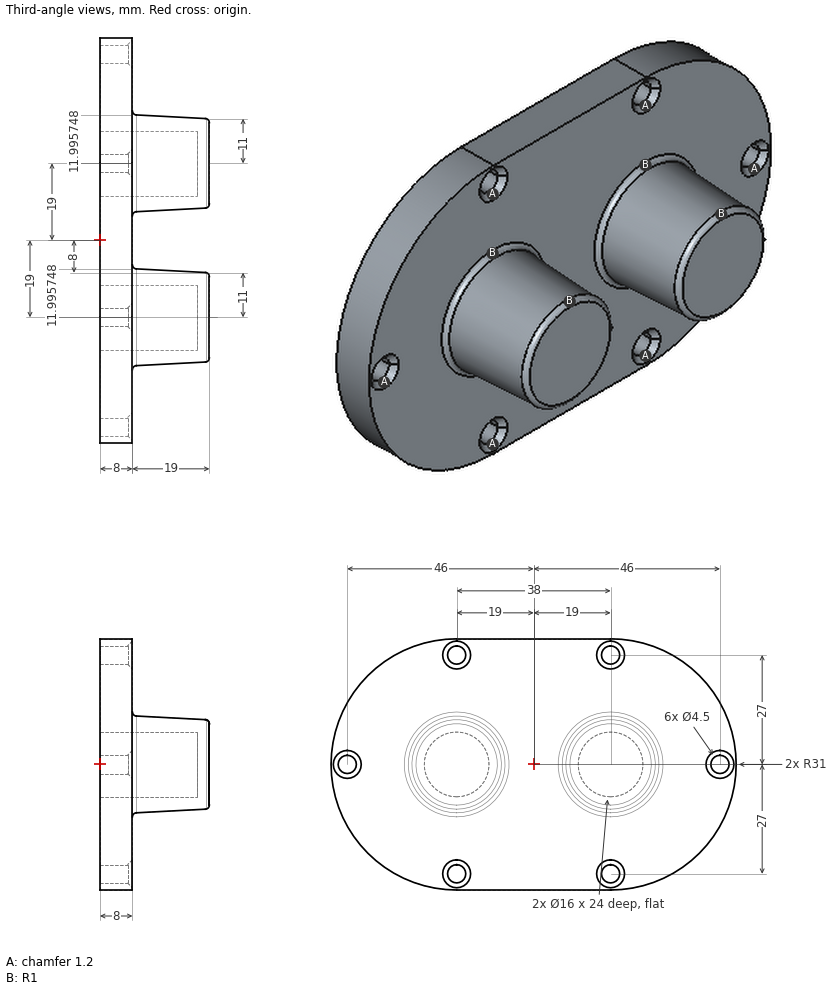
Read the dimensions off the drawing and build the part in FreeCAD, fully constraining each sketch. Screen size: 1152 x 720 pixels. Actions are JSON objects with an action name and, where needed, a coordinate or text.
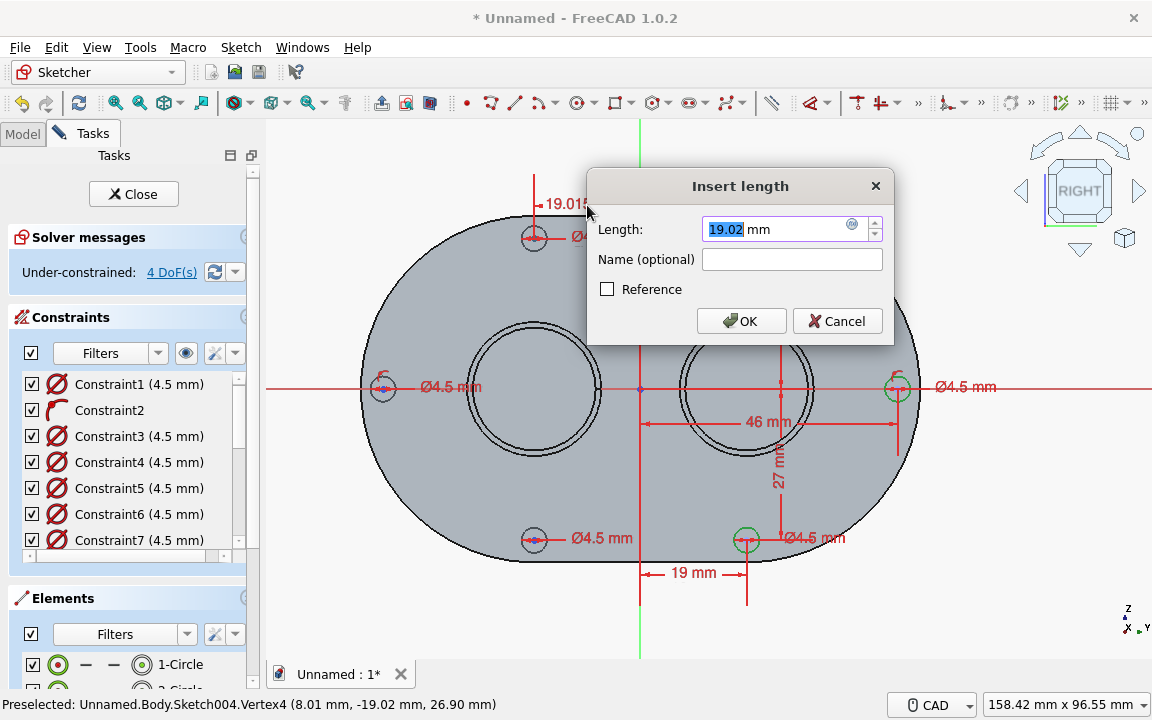
{"action": "type", "text": "19"}
{"action": "key", "text": "Return"}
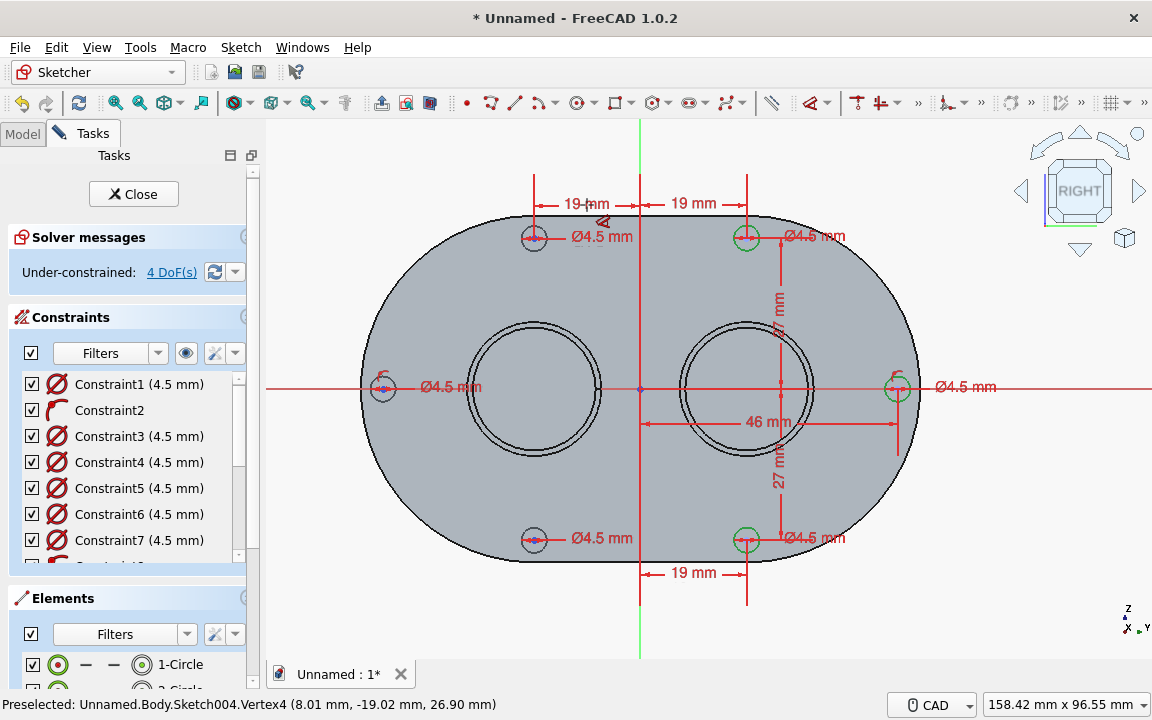
{"action": "left_click", "coordinate": [534, 239]}
{"action": "left_click", "coordinate": [500, 314]}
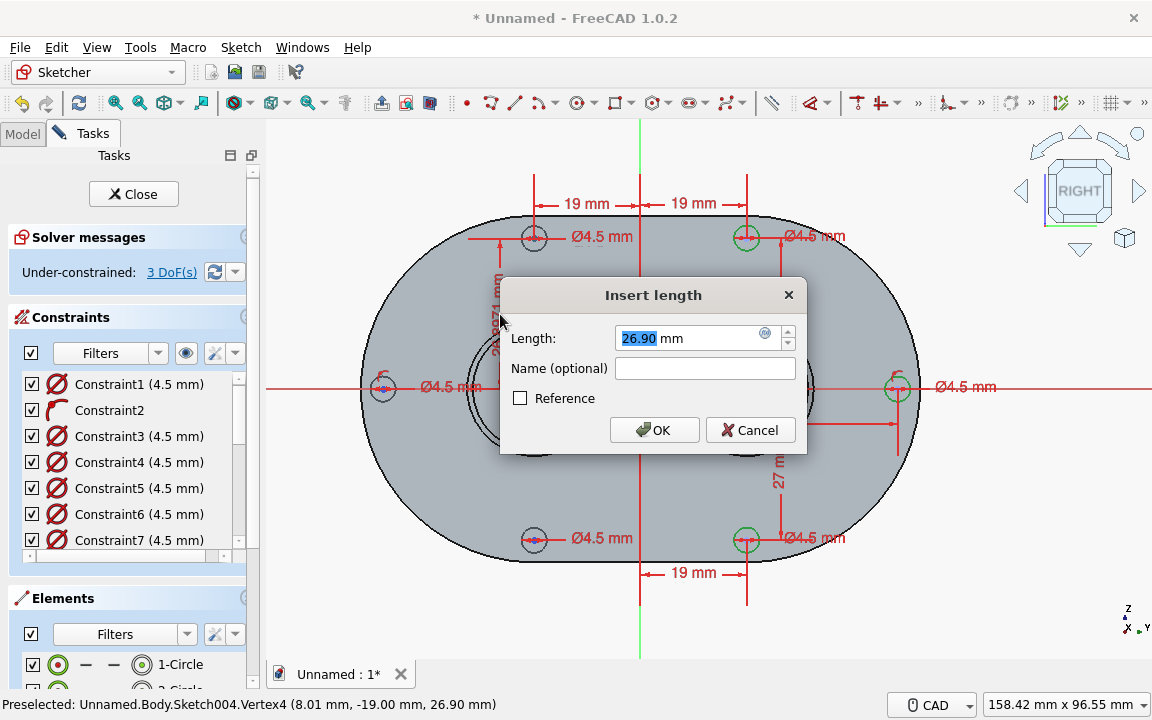
{"action": "type", "text": "27"}
{"action": "key", "text": "Return"}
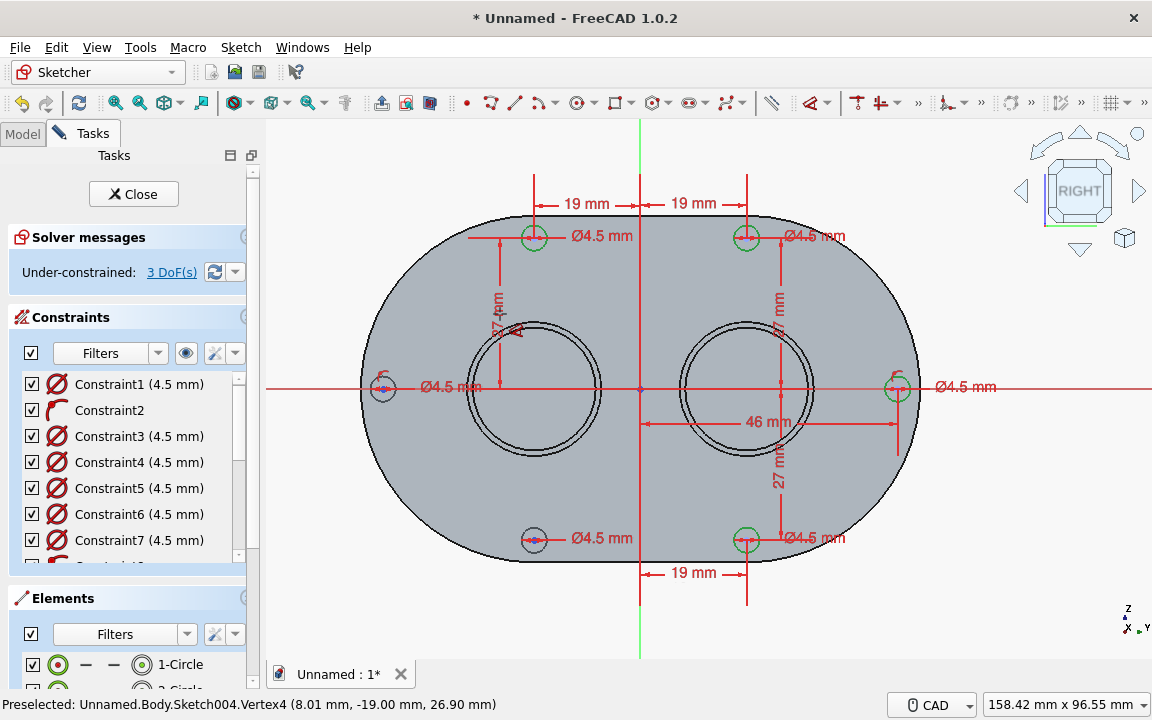
{"action": "left_click", "coordinate": [534, 540]}
{"action": "left_click", "coordinate": [587, 574]}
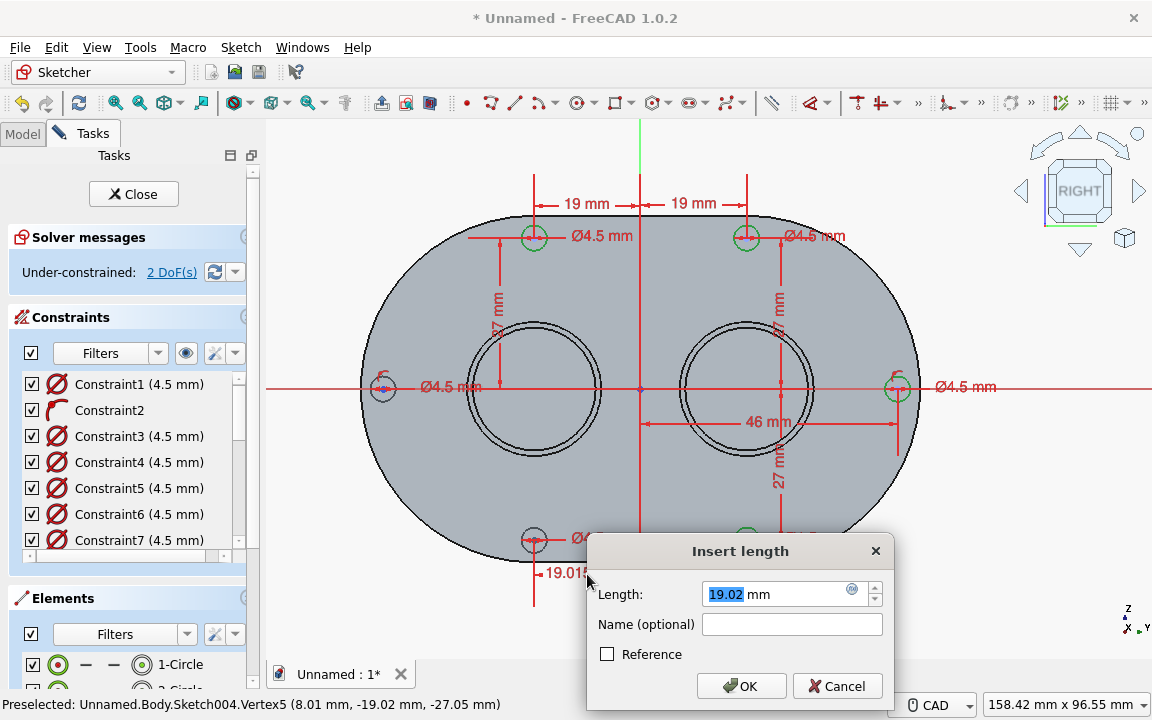
{"action": "type", "text": "19"}
{"action": "key", "text": "Return"}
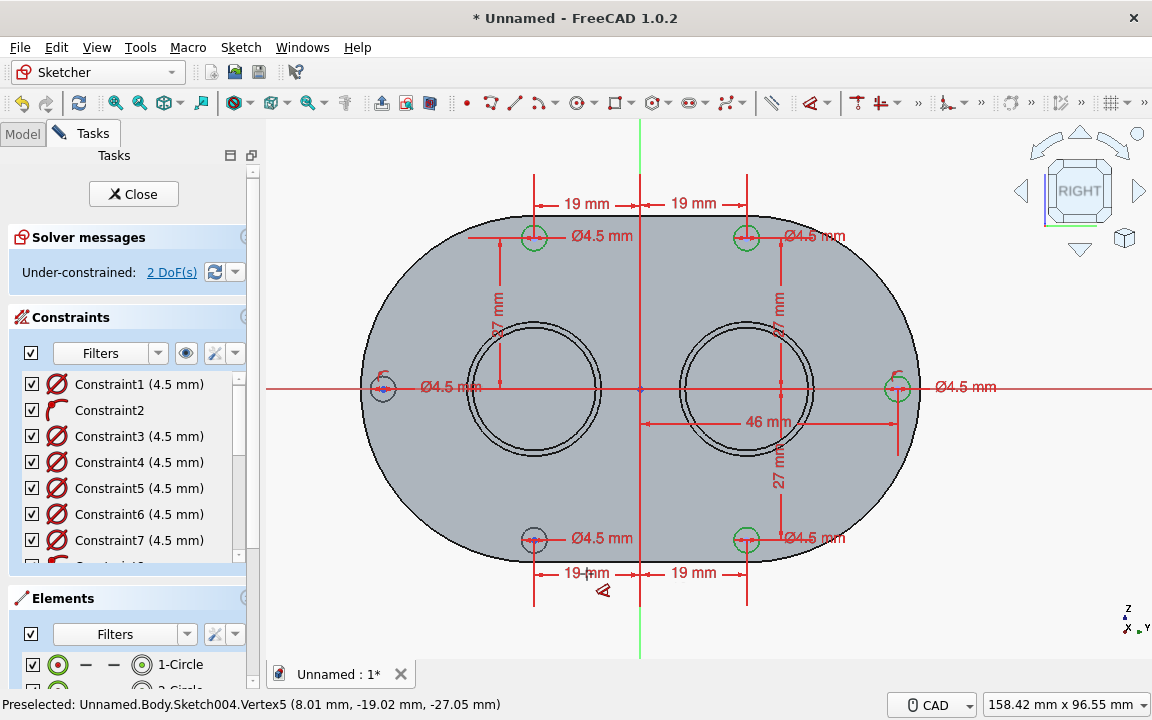
{"action": "left_click", "coordinate": [534, 540]}
{"action": "left_click", "coordinate": [500, 465]}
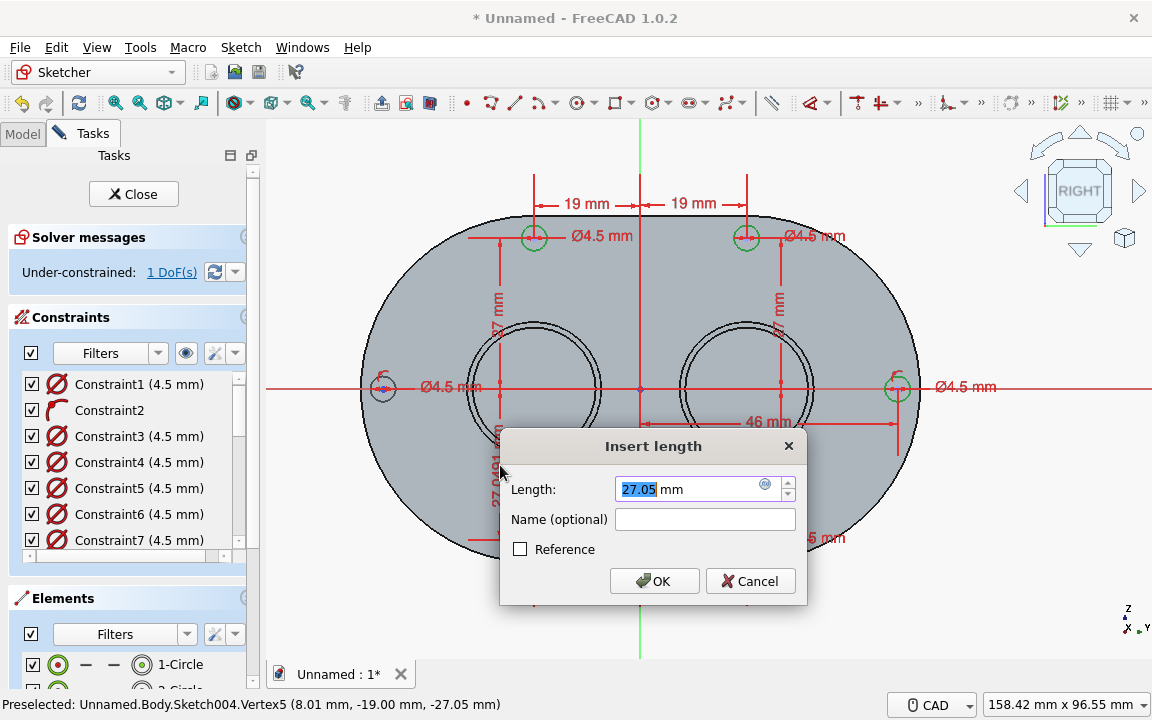
{"action": "type", "text": "27"}
{"action": "key", "text": "Return"}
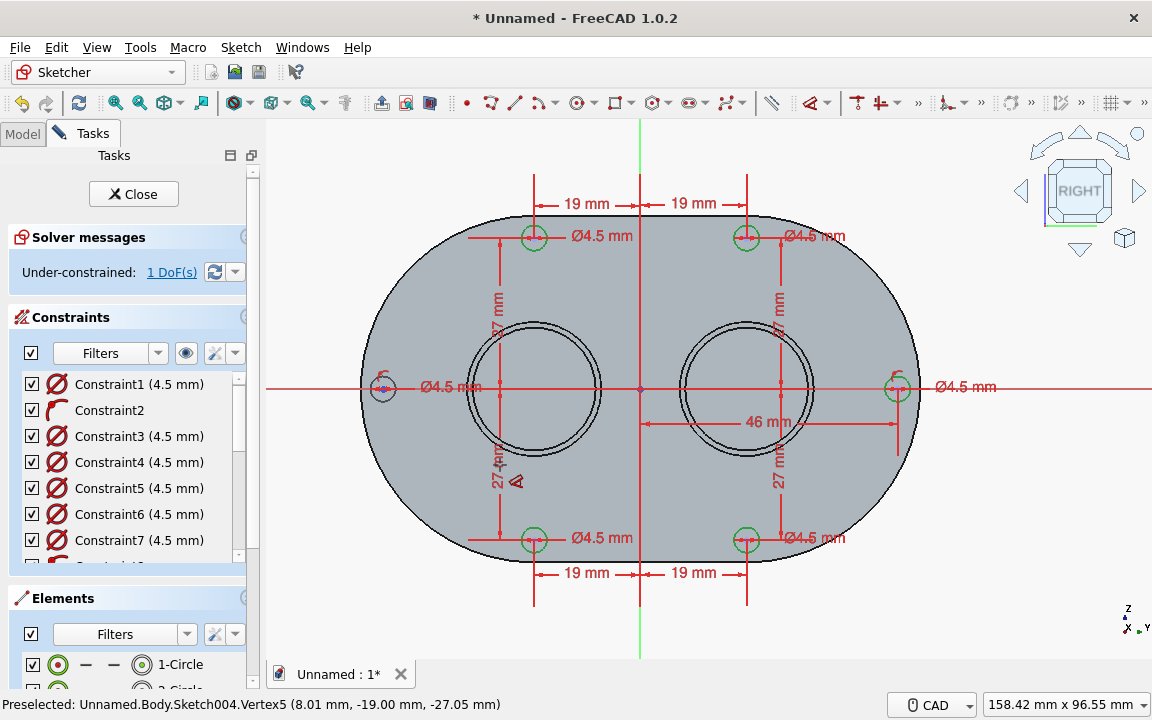
{"action": "left_click", "coordinate": [383, 389]}
{"action": "left_click", "coordinate": [512, 423]}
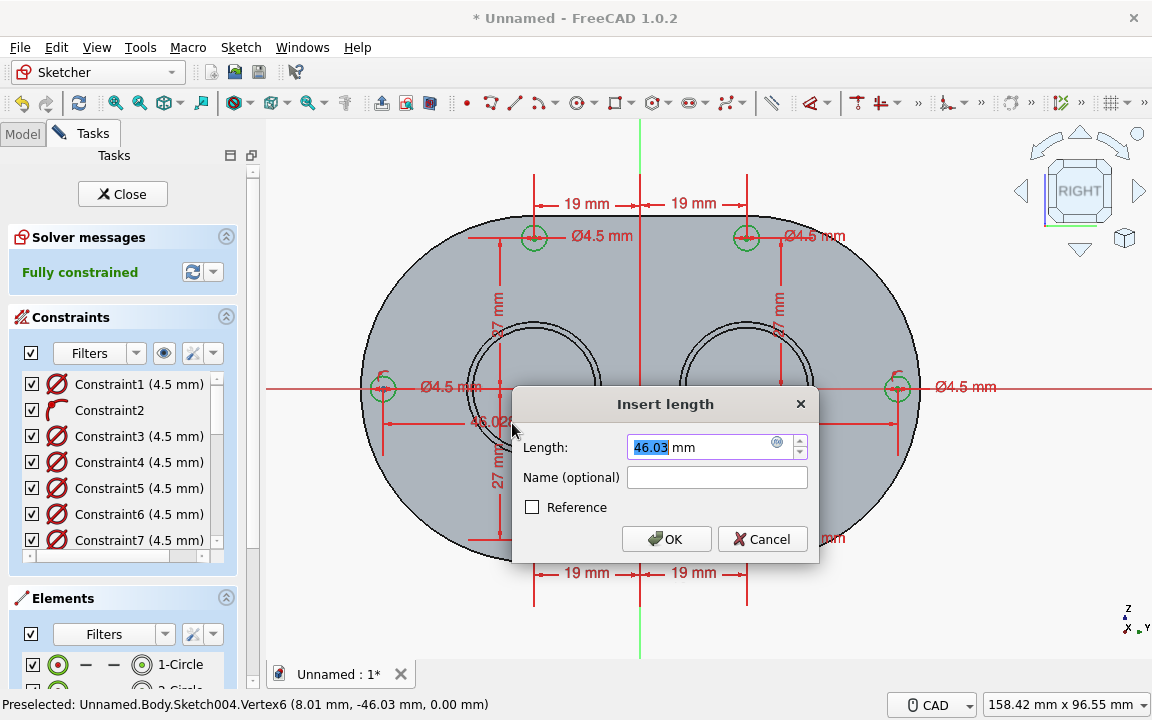
{"action": "type", "text": "46"}
{"action": "key", "text": "Return"}
{"action": "key", "text": "Escape"}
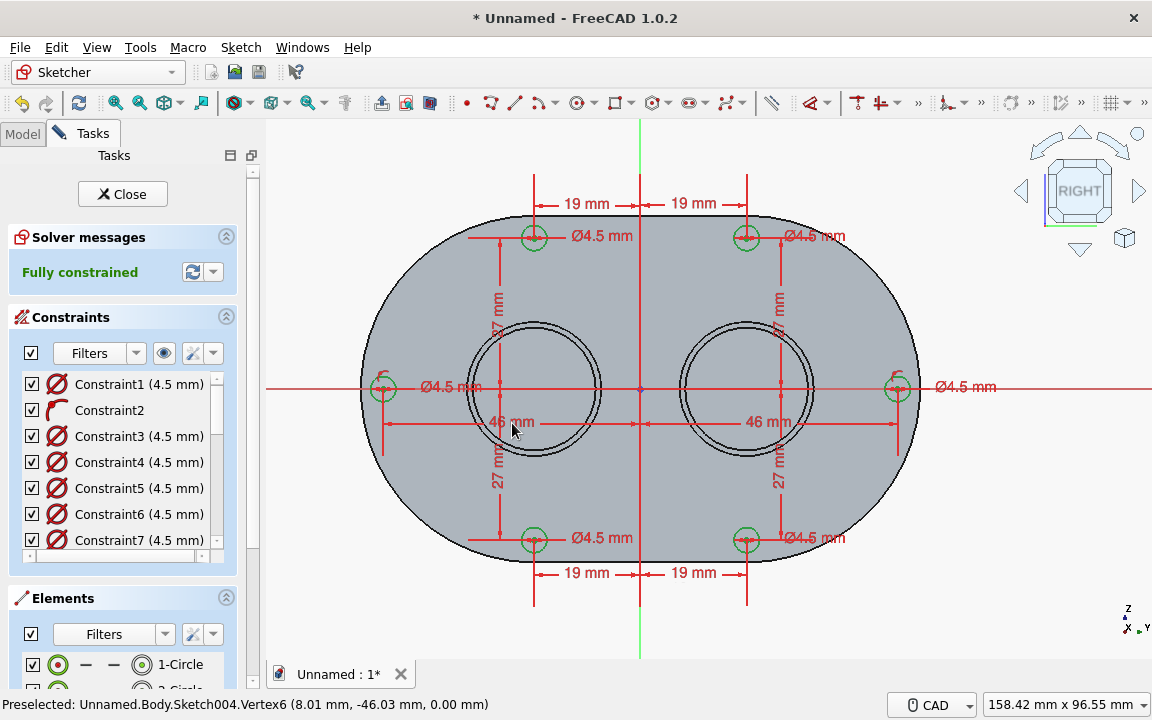
{"action": "left_click", "coordinate": [123, 194]}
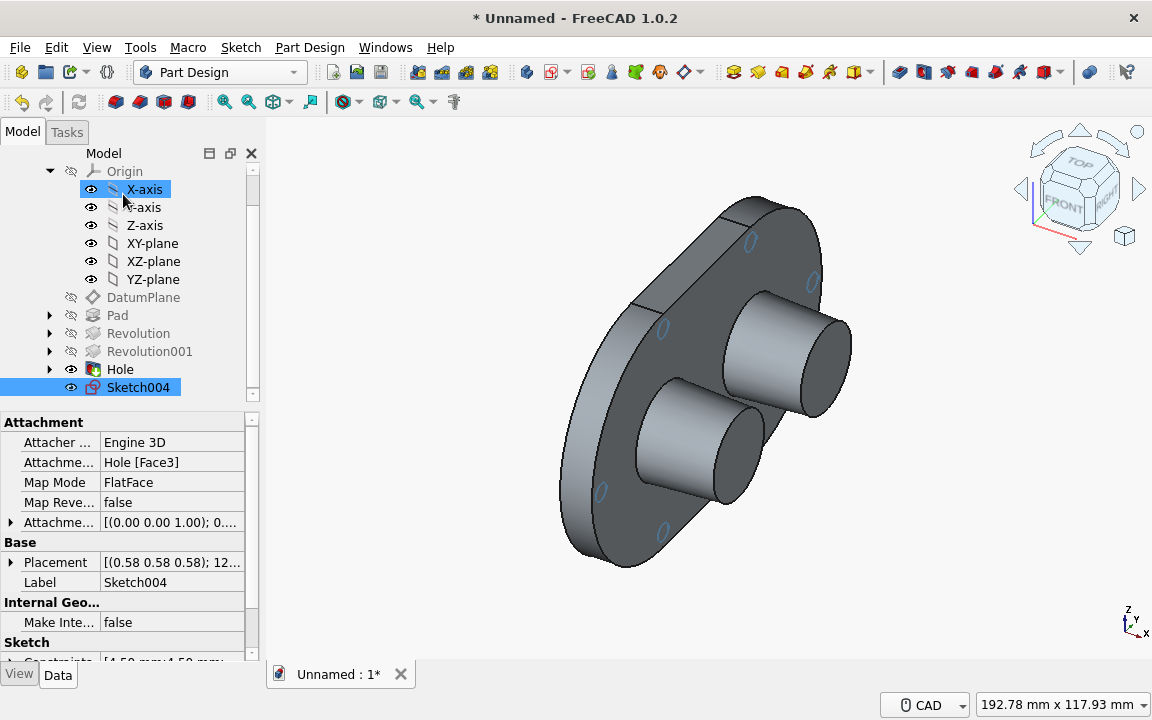
{"action": "left_click", "coordinate": [900, 72]}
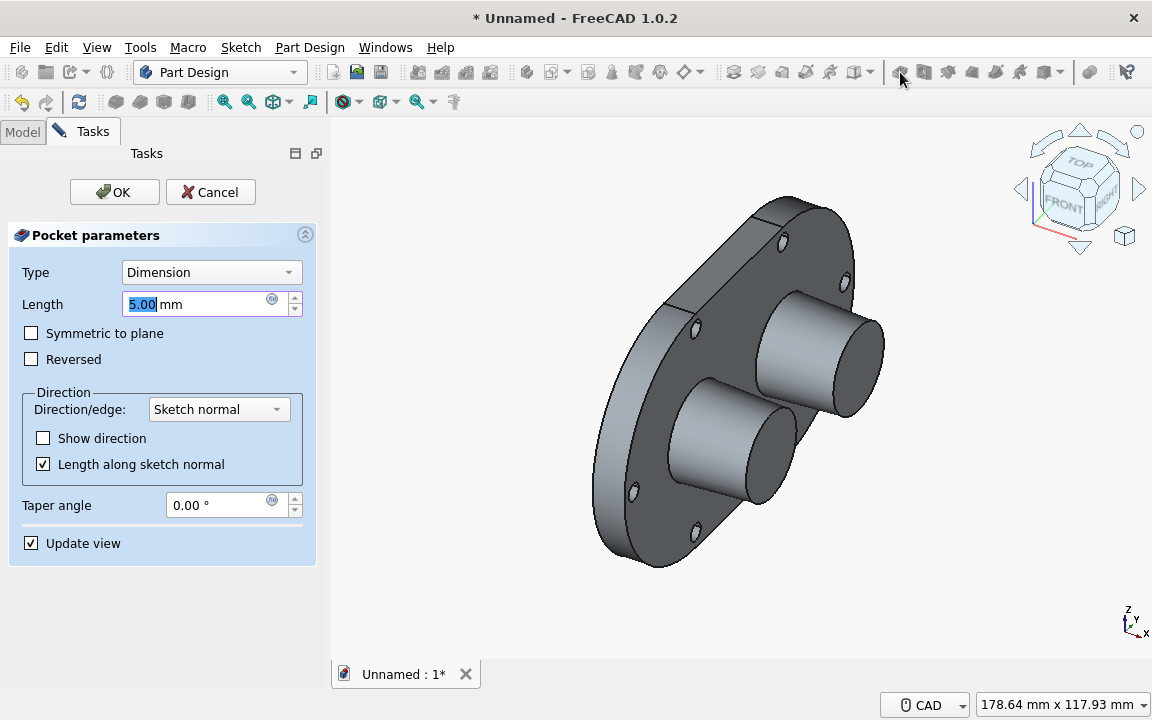
{"action": "left_click", "coordinate": [212, 272]}